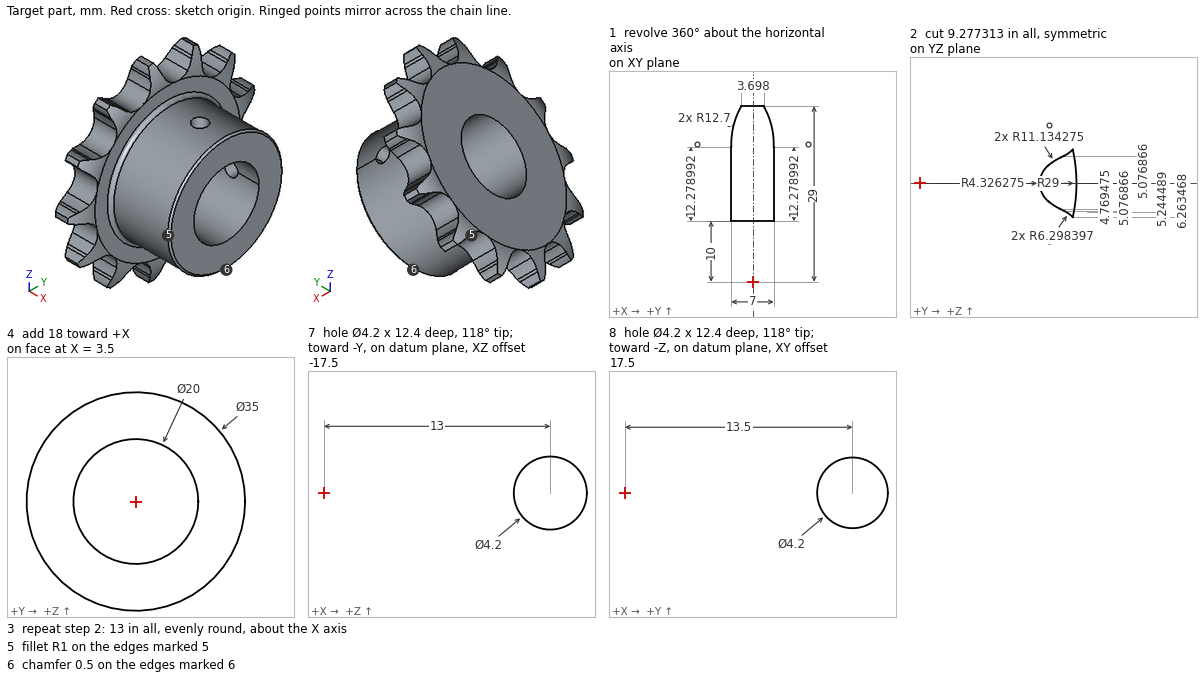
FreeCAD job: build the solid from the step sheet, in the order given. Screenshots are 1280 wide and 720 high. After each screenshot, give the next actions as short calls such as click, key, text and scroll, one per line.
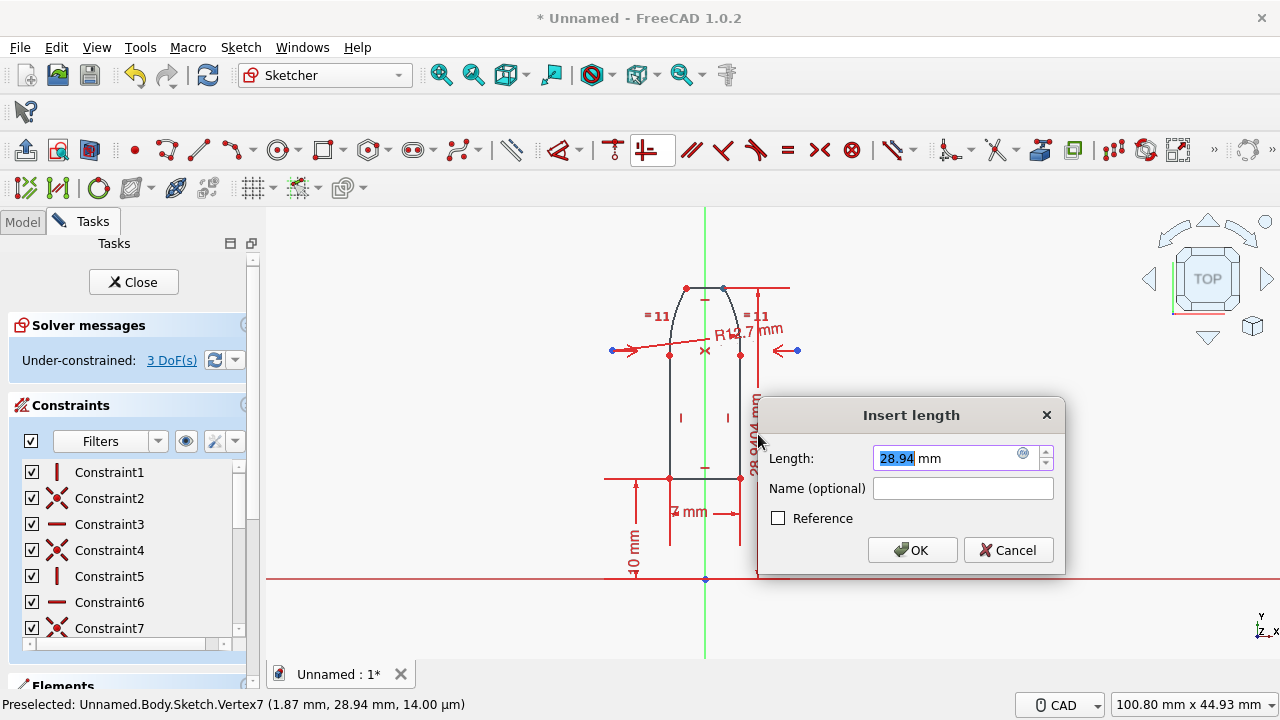
text(29)
key(Return)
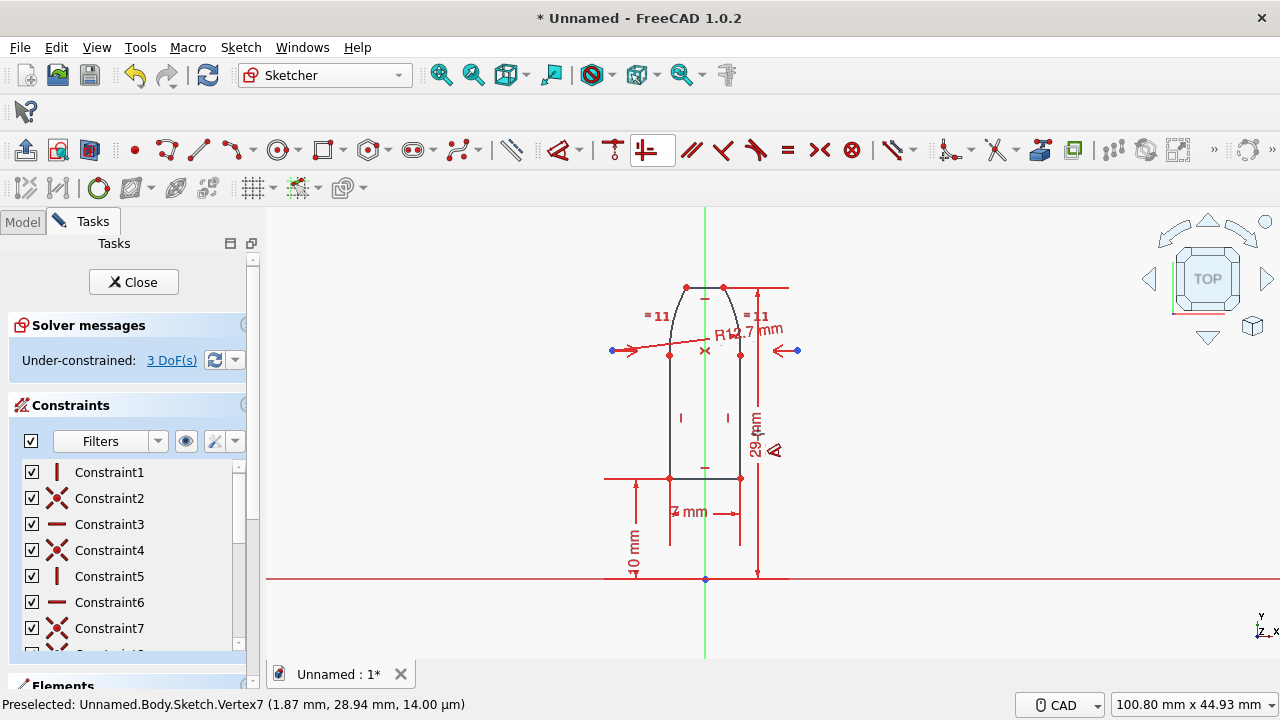
click(709, 288)
click(697, 254)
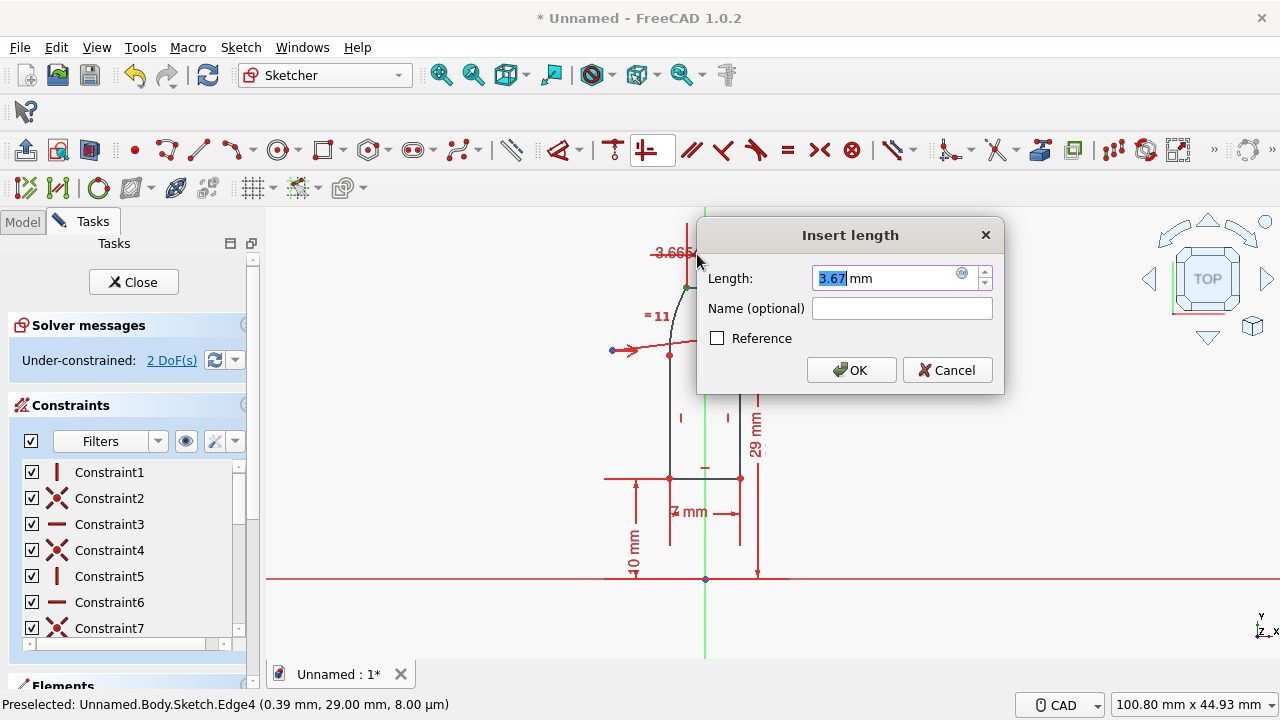
text(3.698)
key(Return)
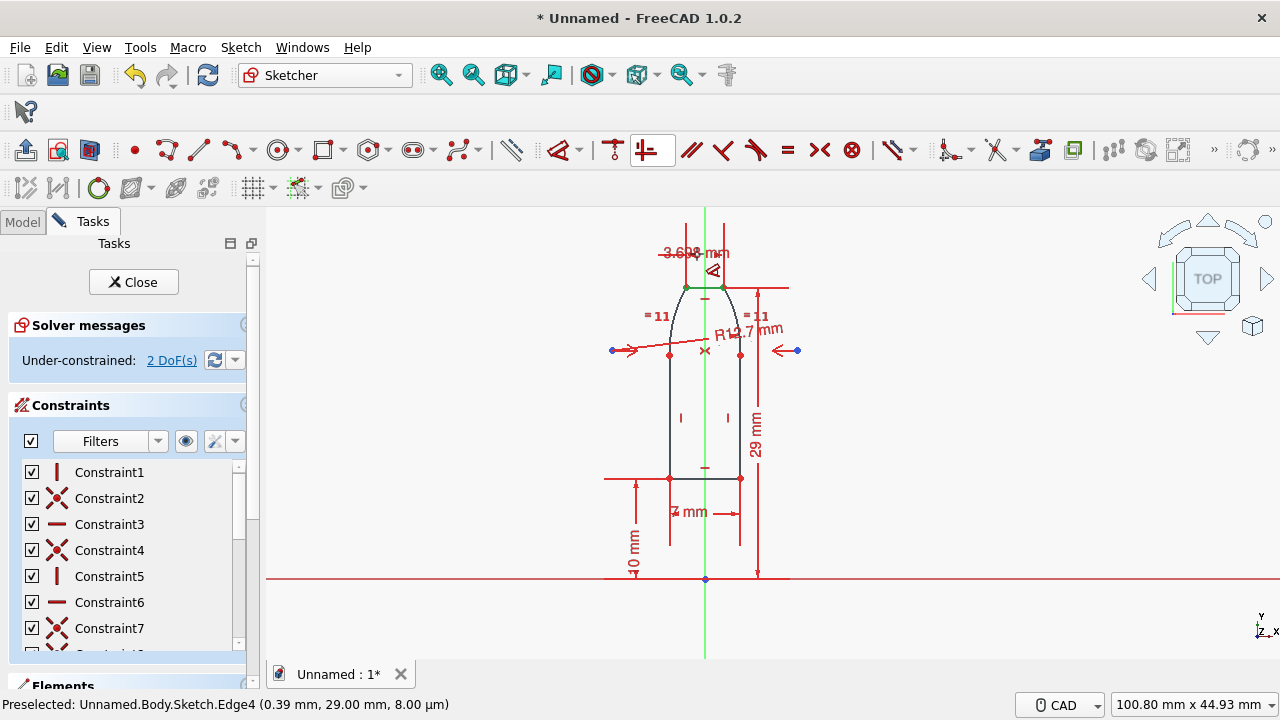
click(670, 393)
click(636, 417)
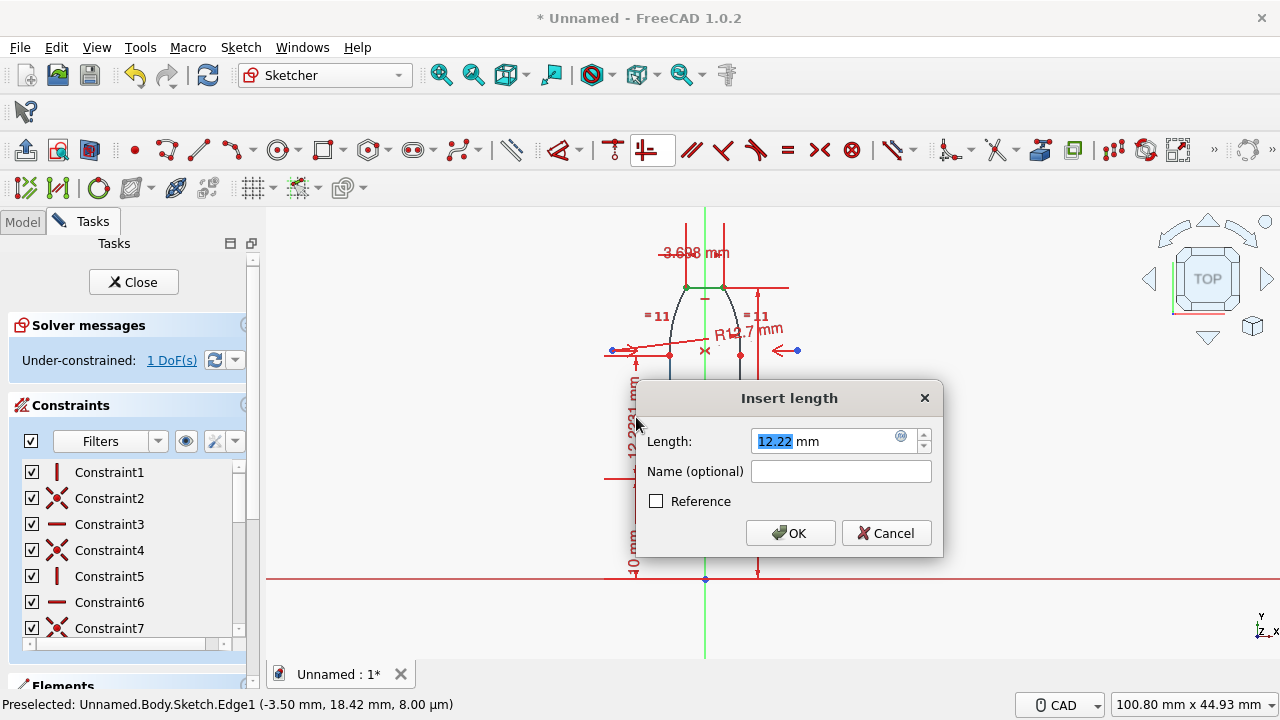
text(12.278992)
key(Return)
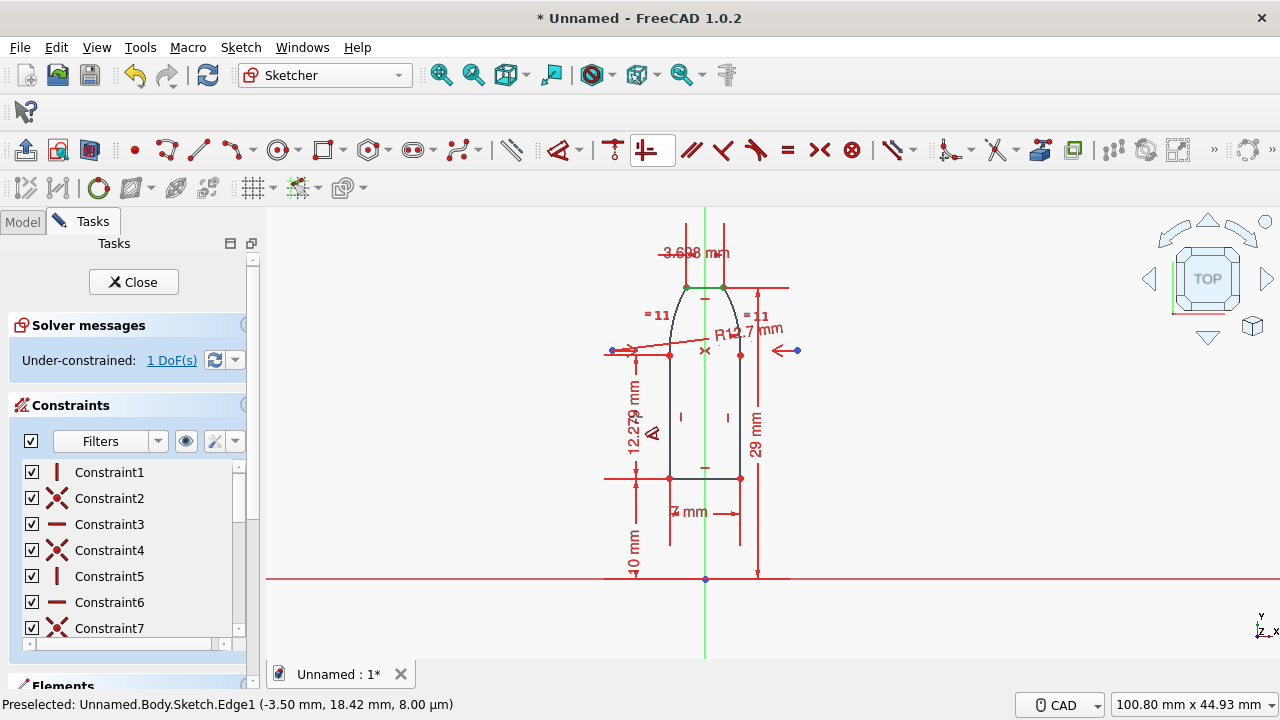
click(740, 442)
click(774, 389)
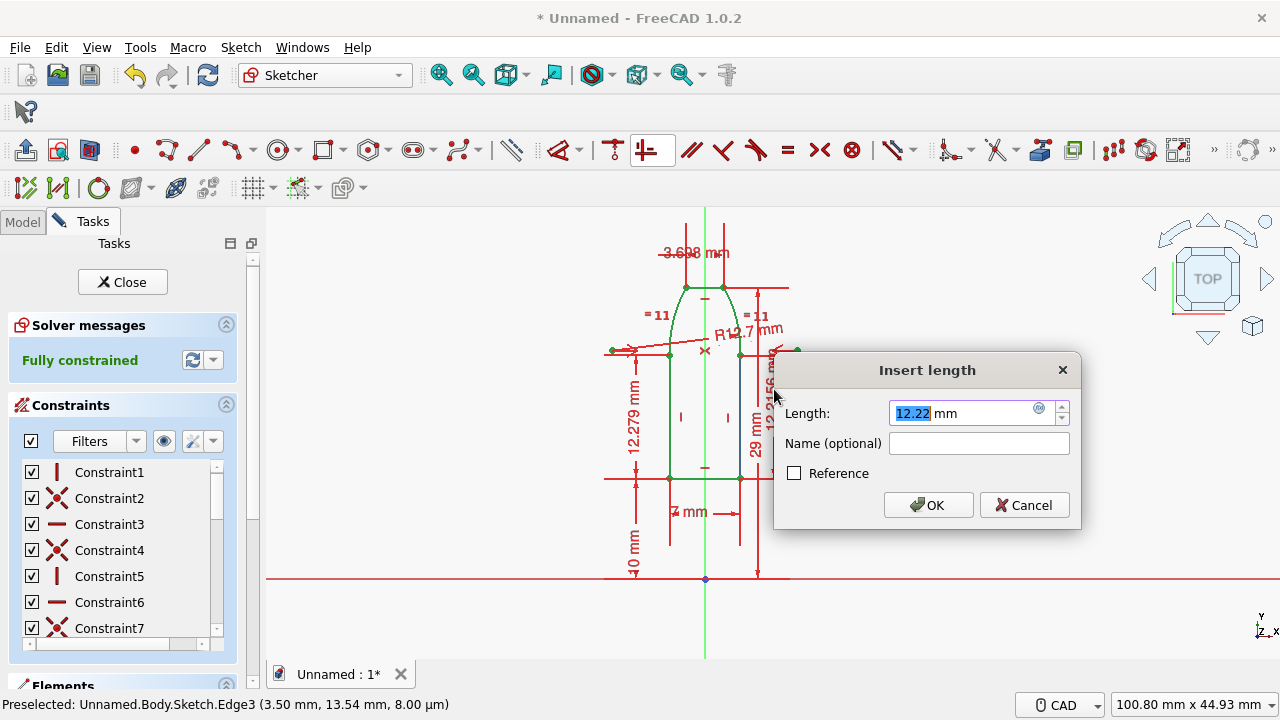
text(12.278992)
key(Return)
key(Escape)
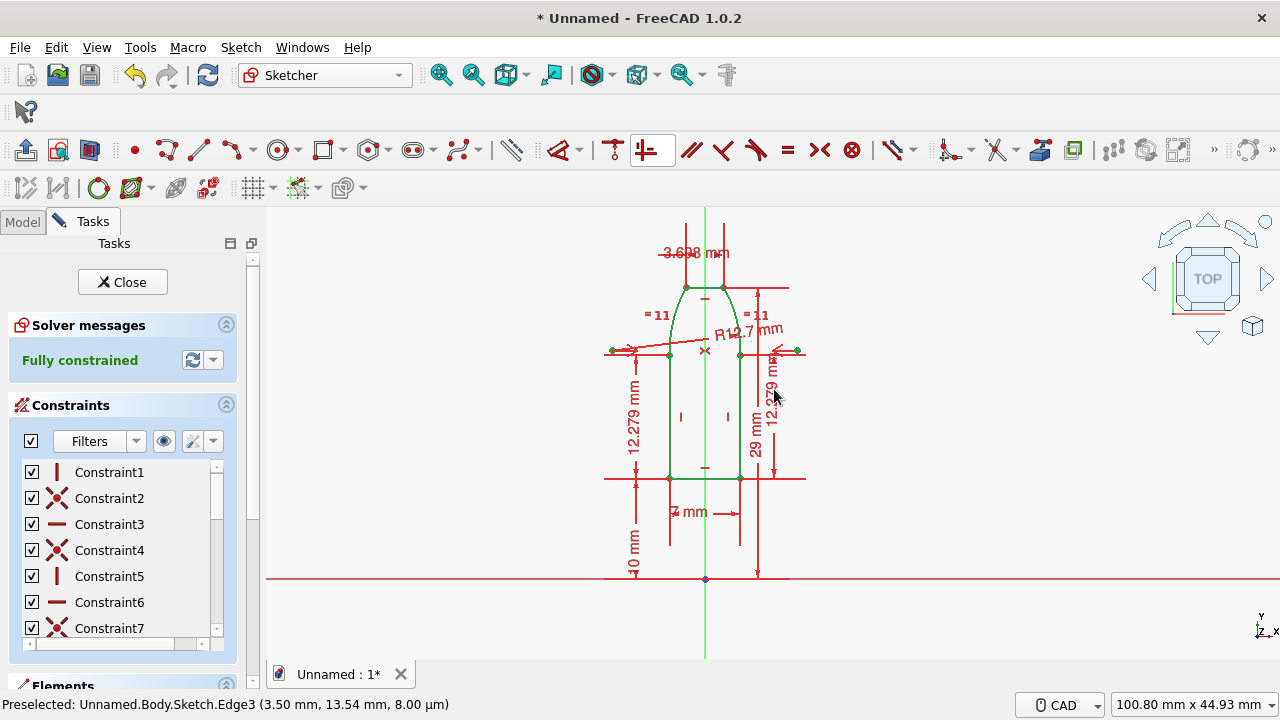
click(123, 282)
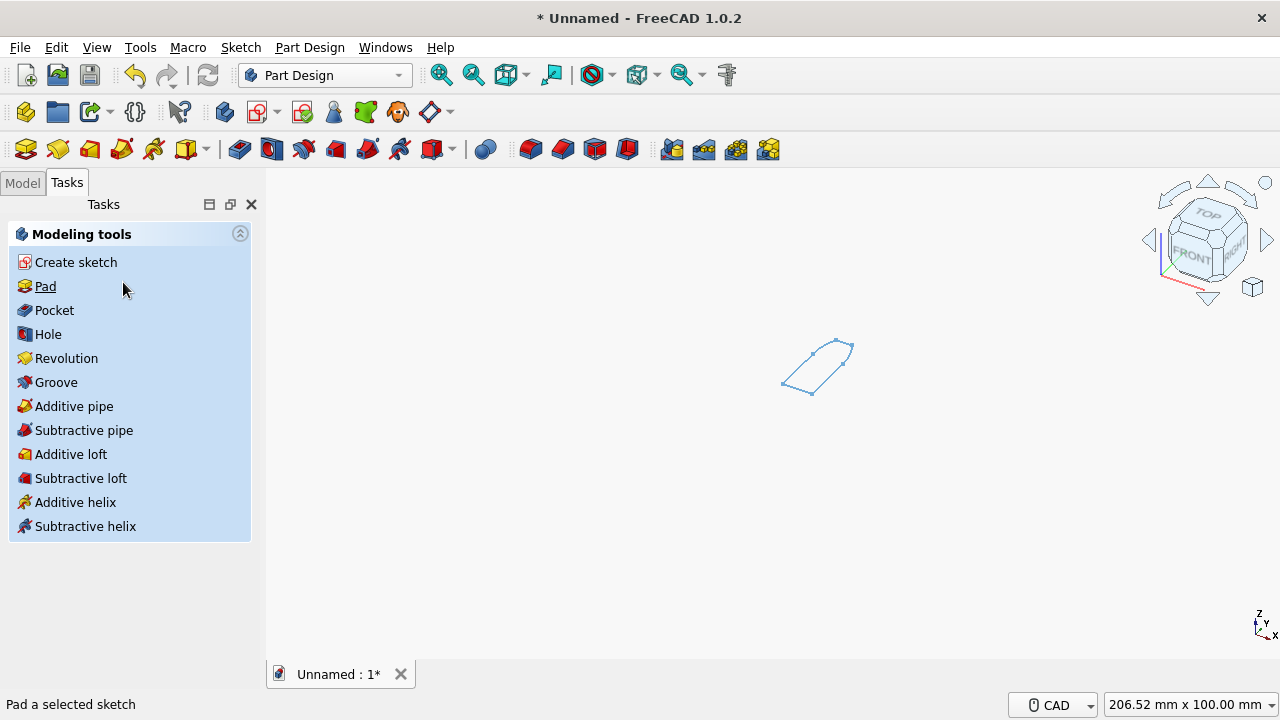
click(58, 150)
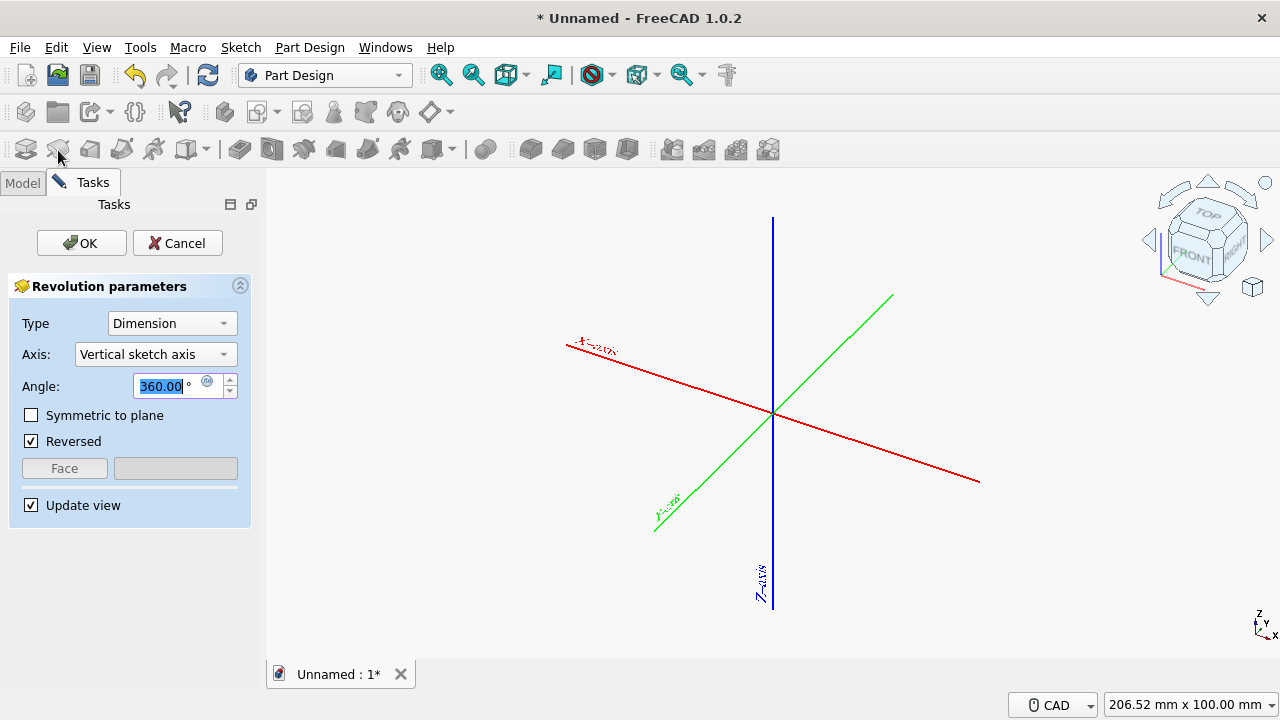
click(156, 354)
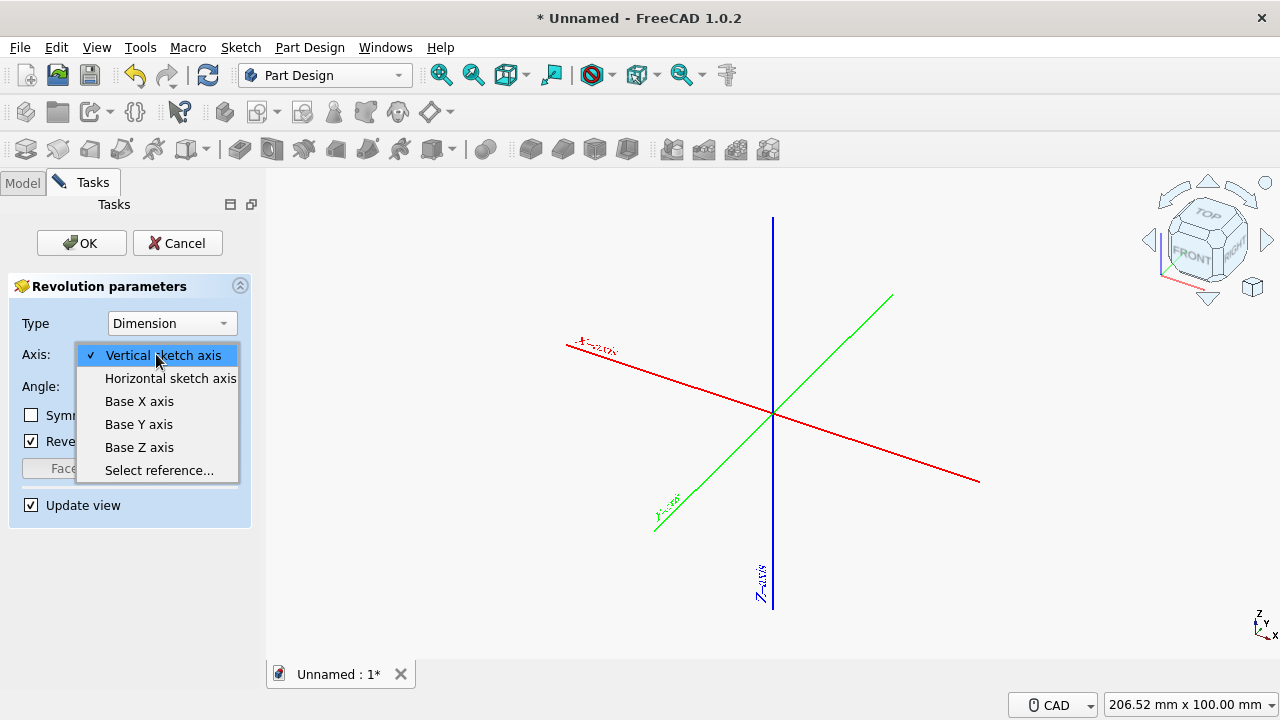
click(156, 378)